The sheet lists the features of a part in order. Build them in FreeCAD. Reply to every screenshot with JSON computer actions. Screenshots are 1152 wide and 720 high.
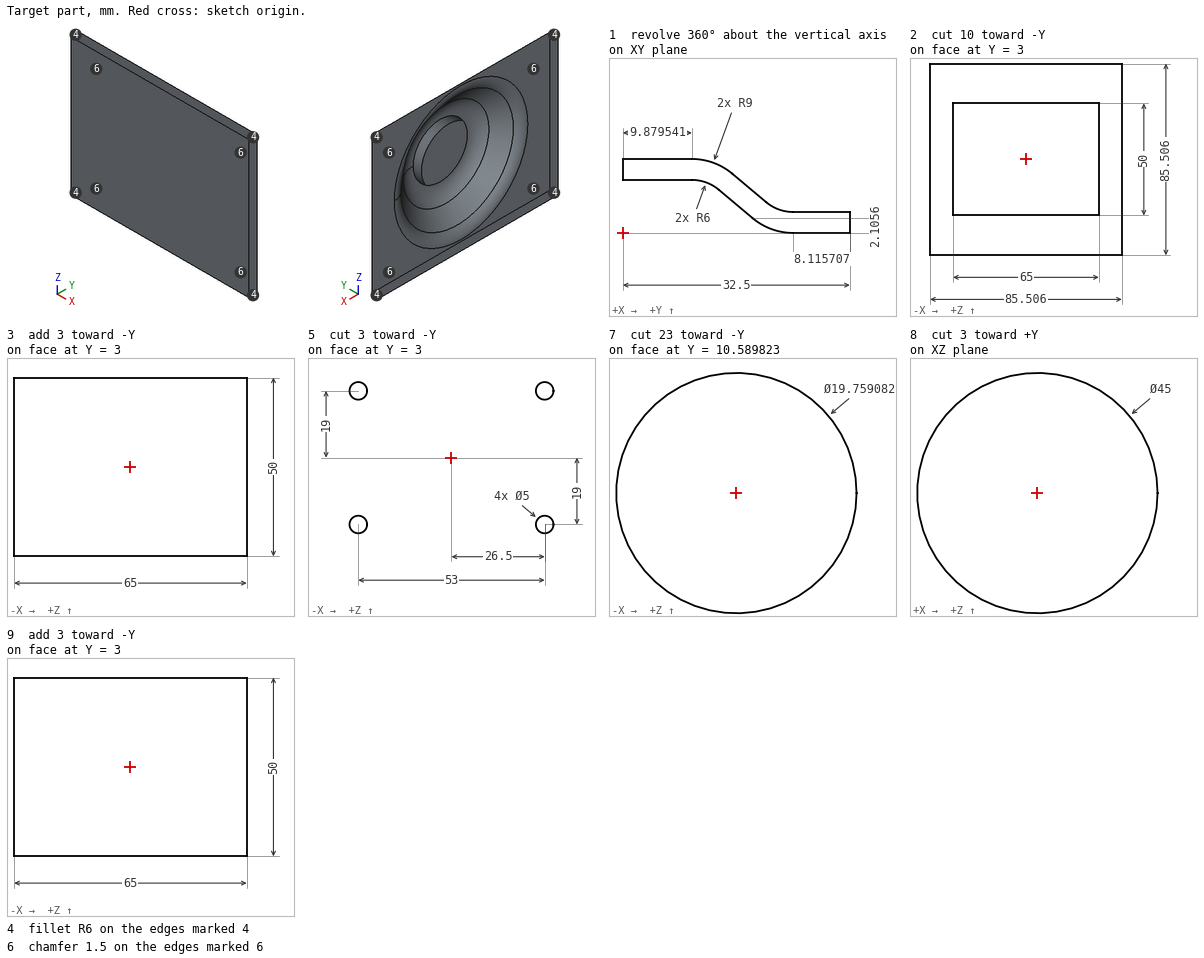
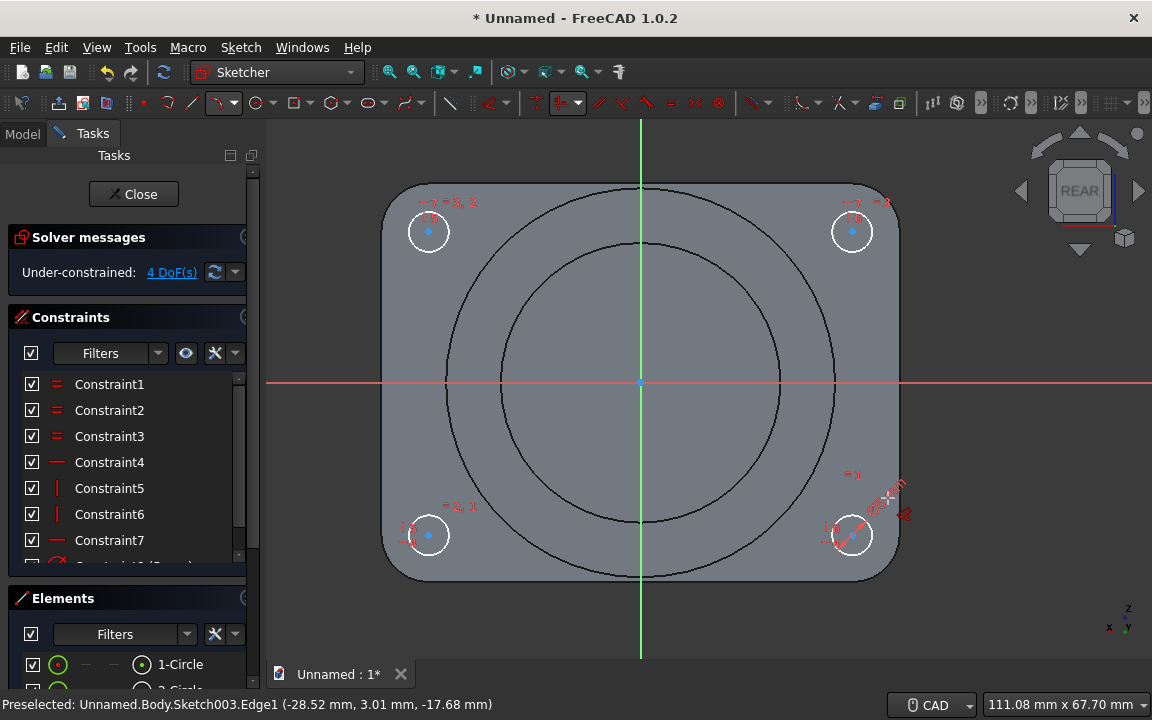
{"action": "left_click", "coordinate": [852, 535]}
{"action": "left_click", "coordinate": [886, 459]}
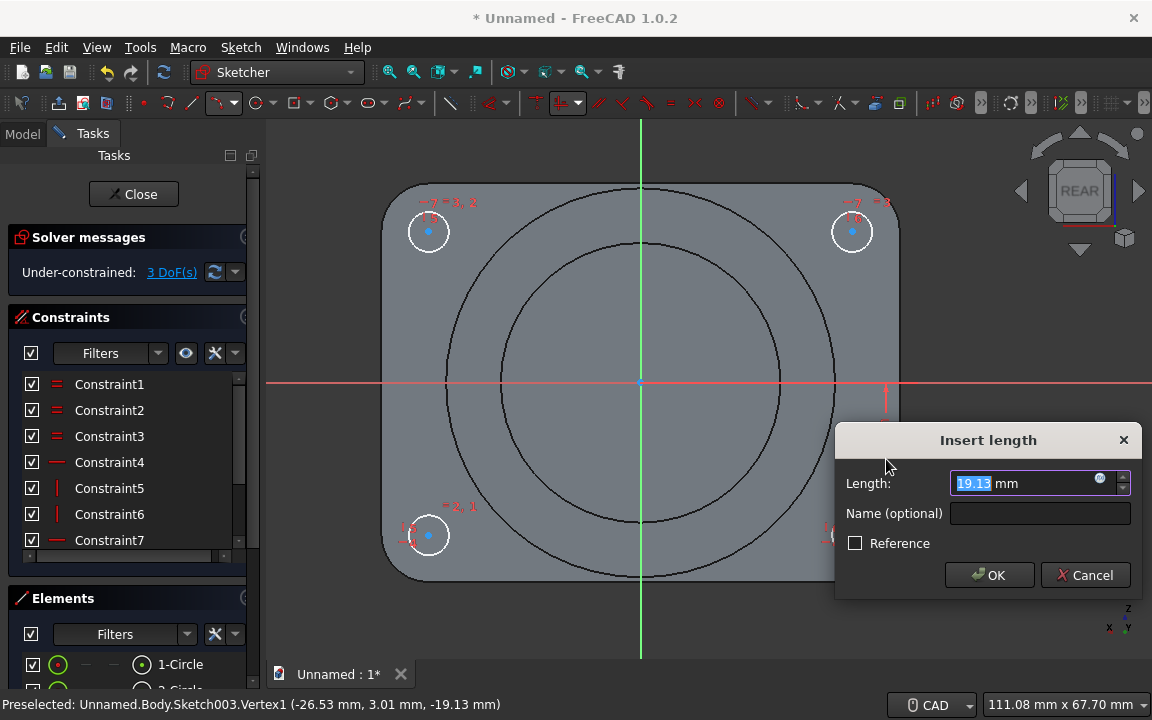
{"action": "type", "text": "19"}
{"action": "key", "text": "Return"}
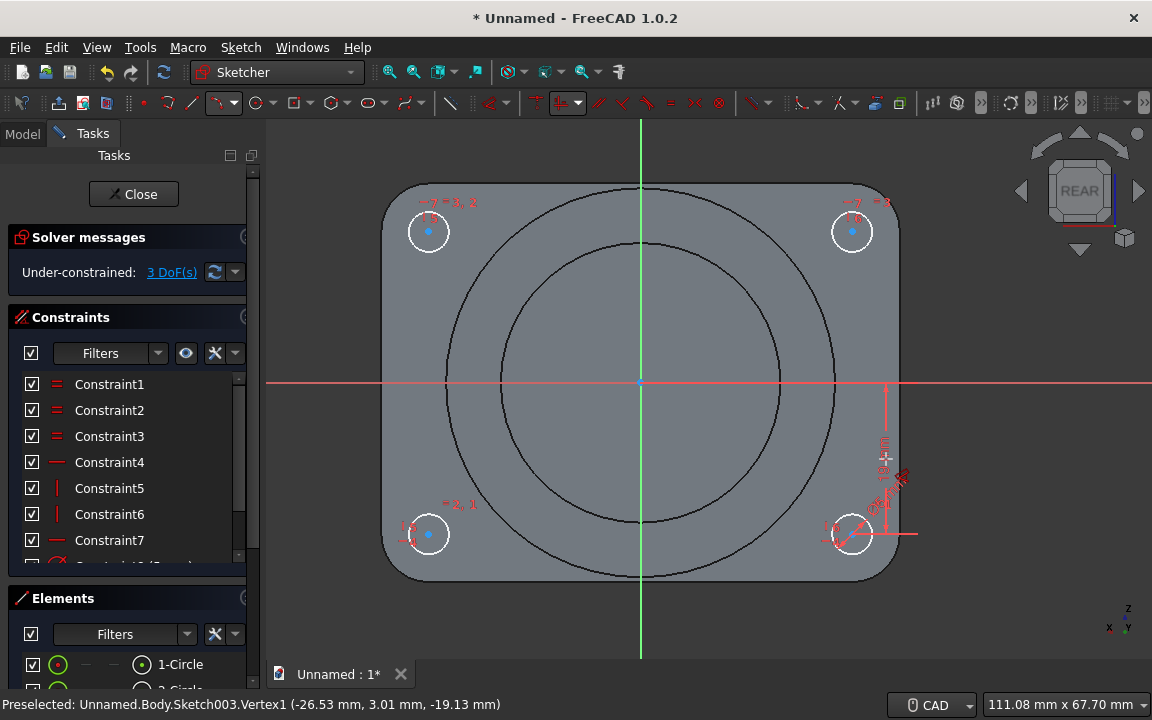
{"action": "left_click", "coordinate": [429, 232]}
{"action": "left_click", "coordinate": [395, 307]}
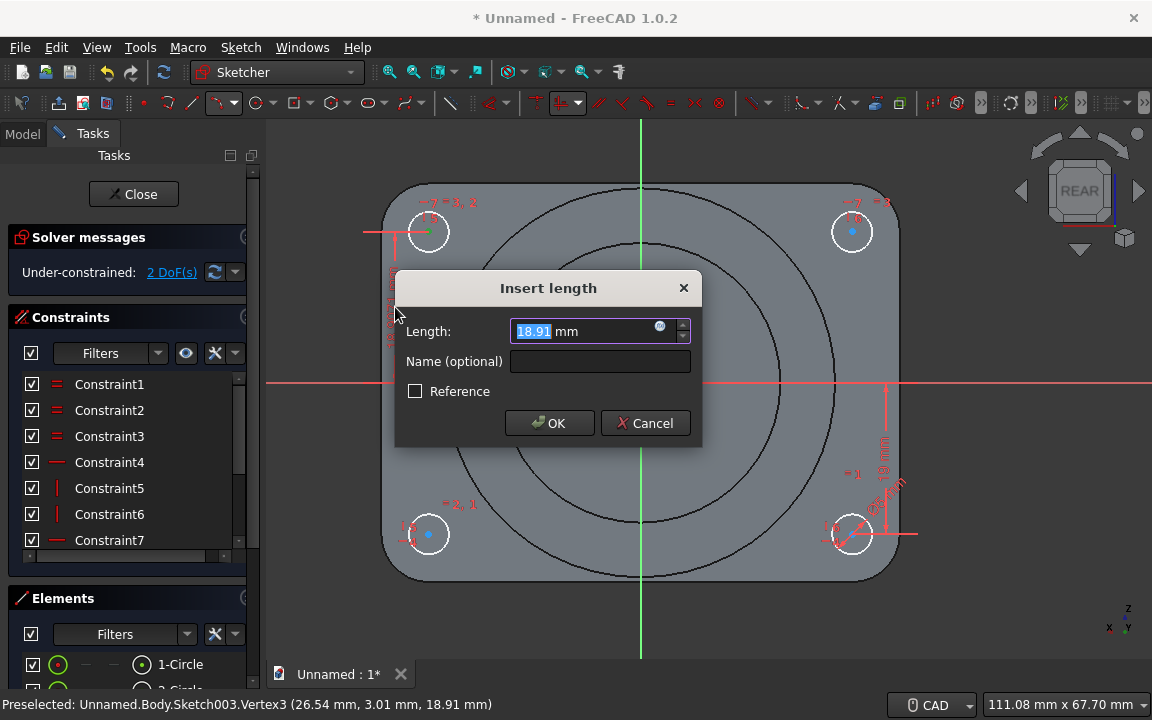
{"action": "type", "text": "19"}
{"action": "key", "text": "Return"}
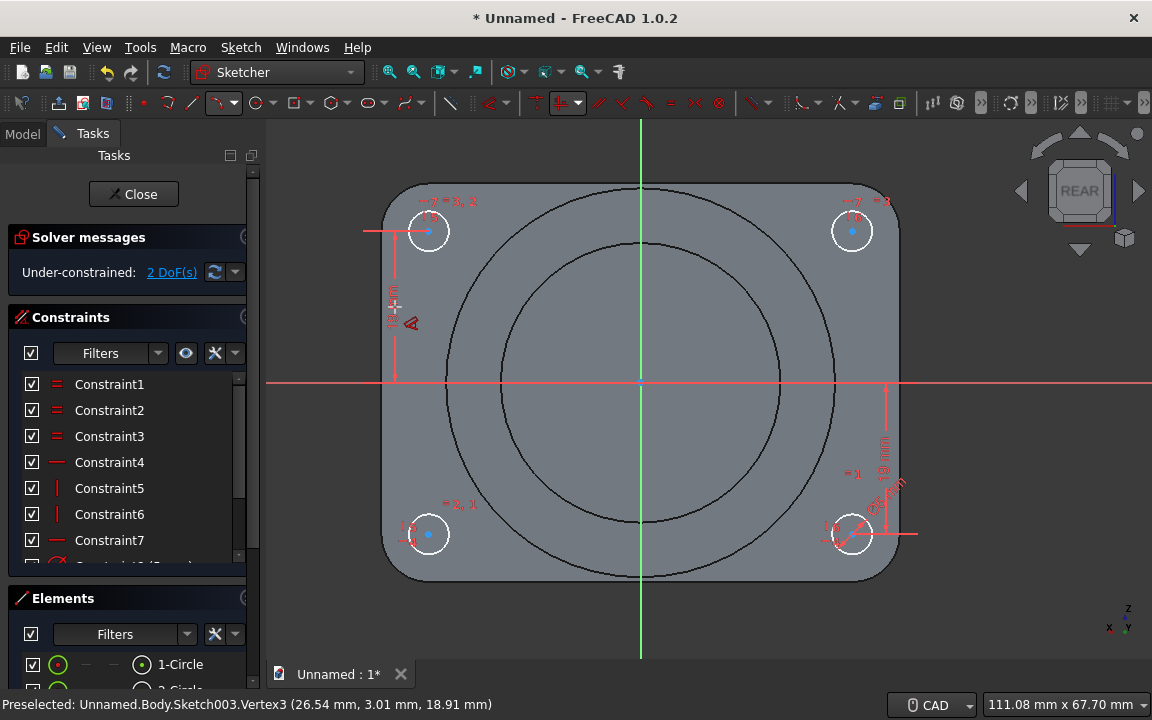
{"action": "left_click", "coordinate": [852, 534]}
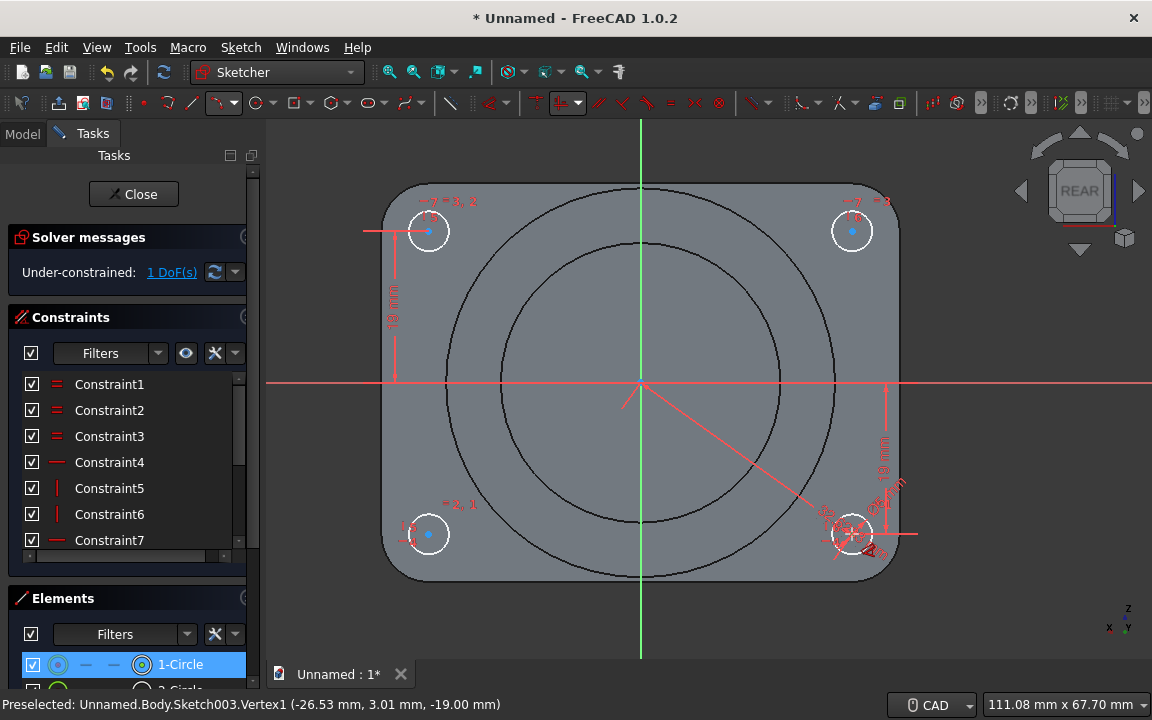
{"action": "left_click", "coordinate": [429, 534]}
{"action": "left_click", "coordinate": [543, 568]}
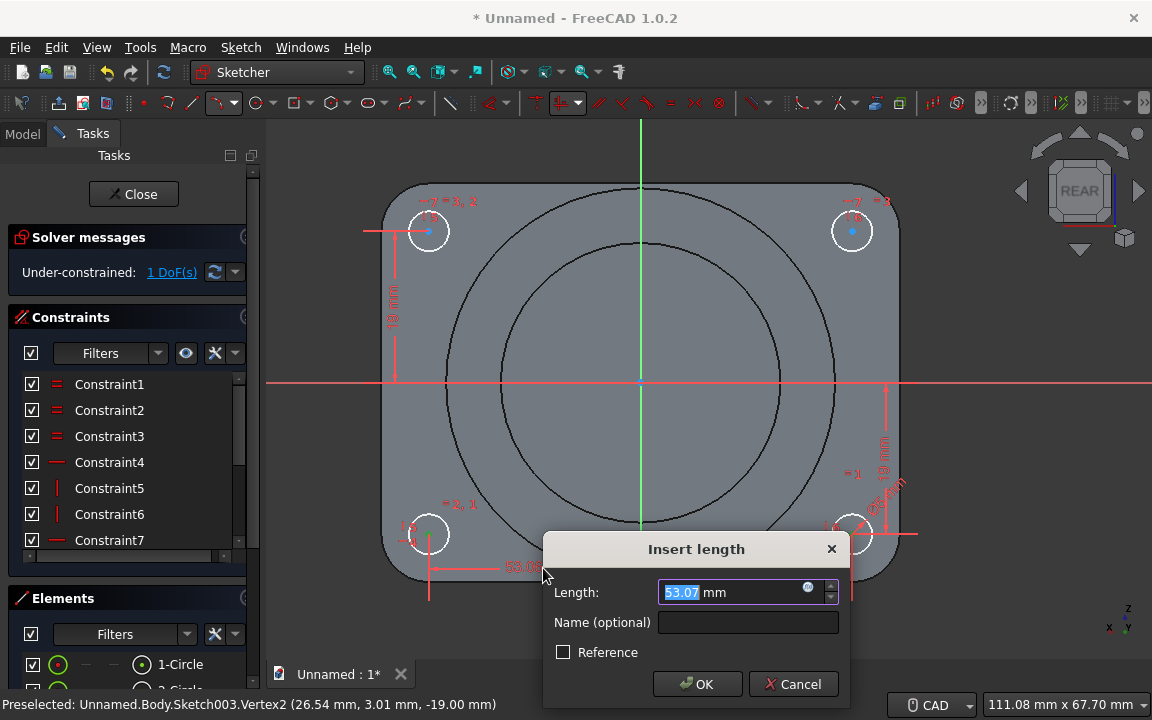
{"action": "type", "text": "53"}
{"action": "key", "text": "Return"}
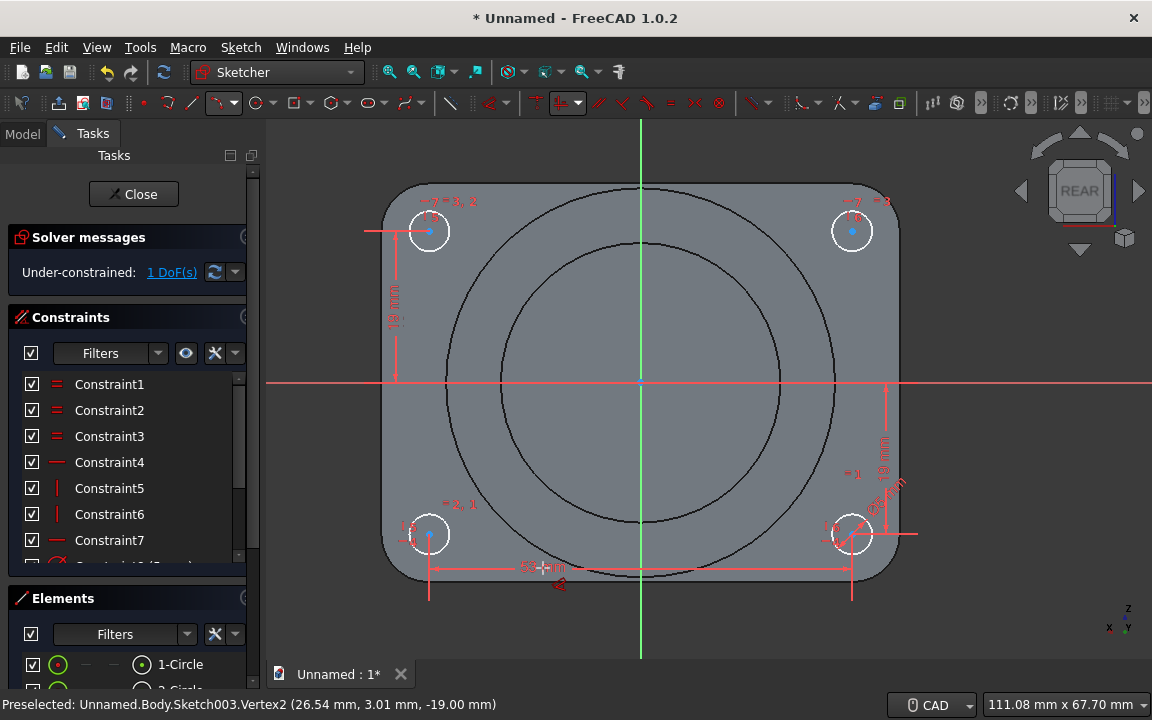
{"action": "left_click", "coordinate": [852, 534]}
{"action": "left_click", "coordinate": [746, 568]}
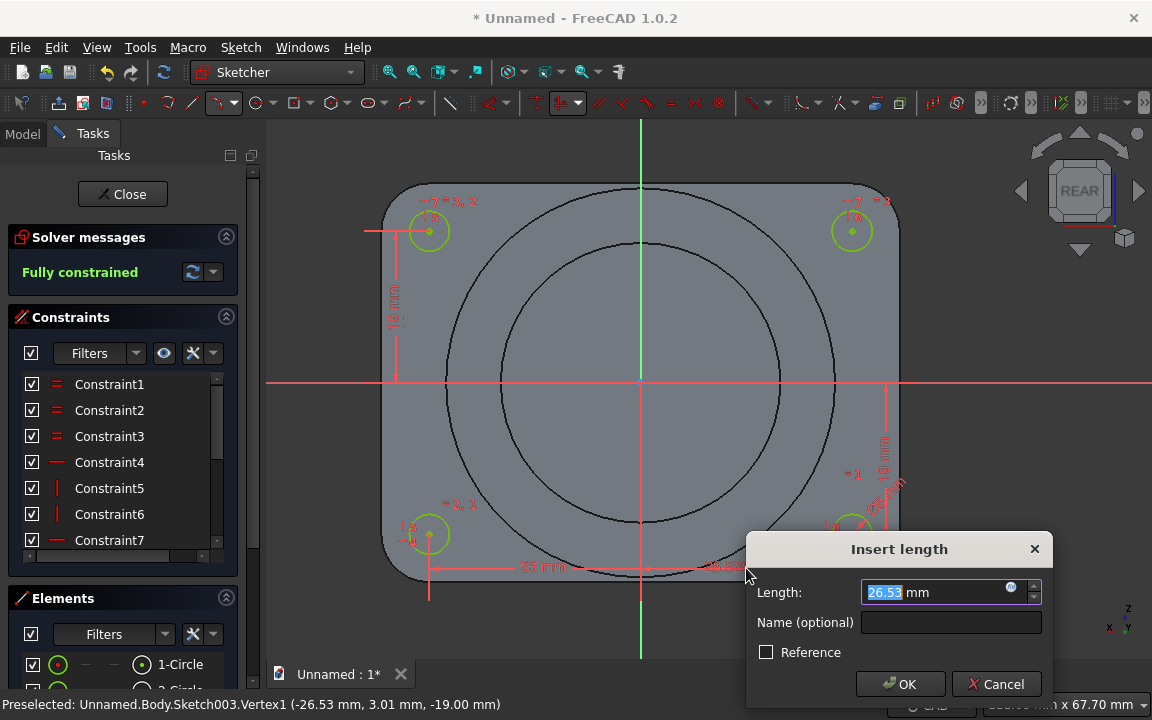
{"action": "type", "text": "26.5"}
{"action": "key", "text": "Return"}
{"action": "key", "text": "Escape"}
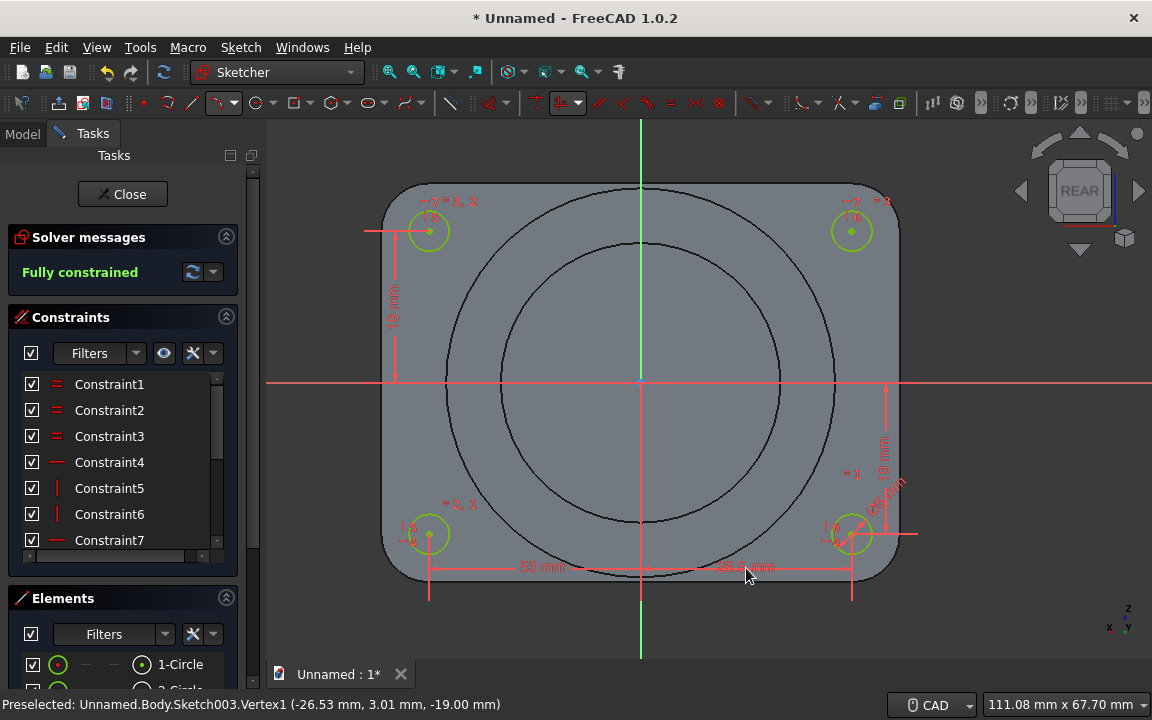
{"action": "left_click", "coordinate": [123, 194]}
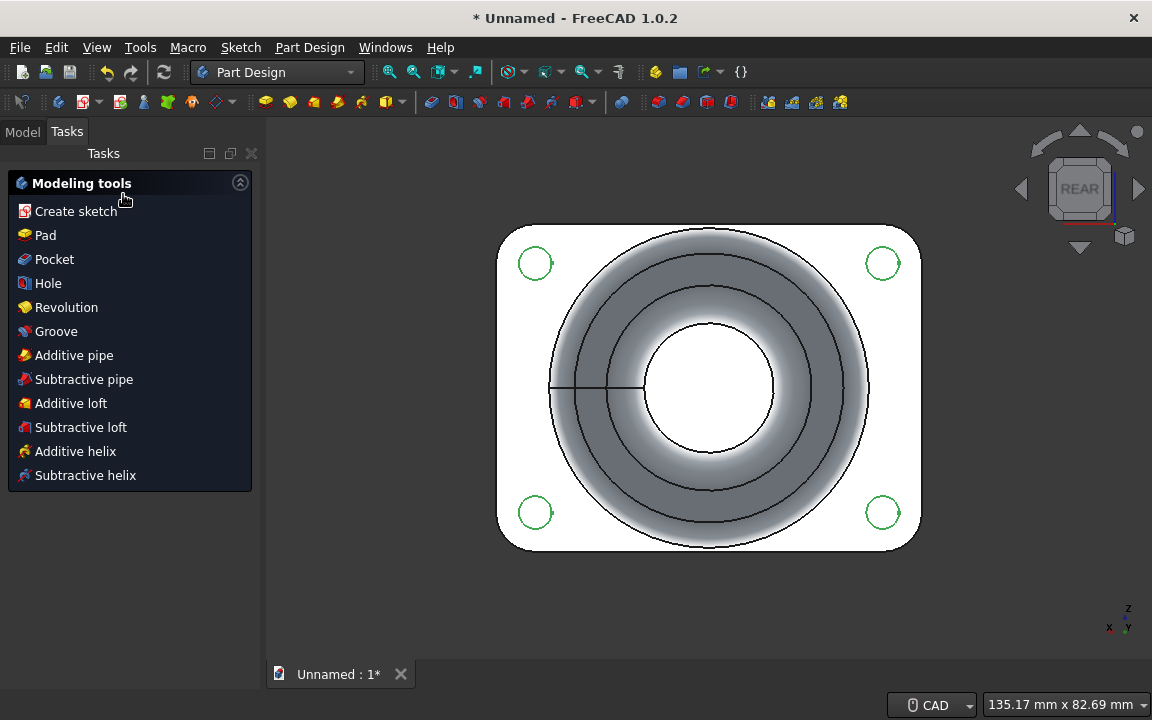
{"action": "left_click", "coordinate": [432, 102]}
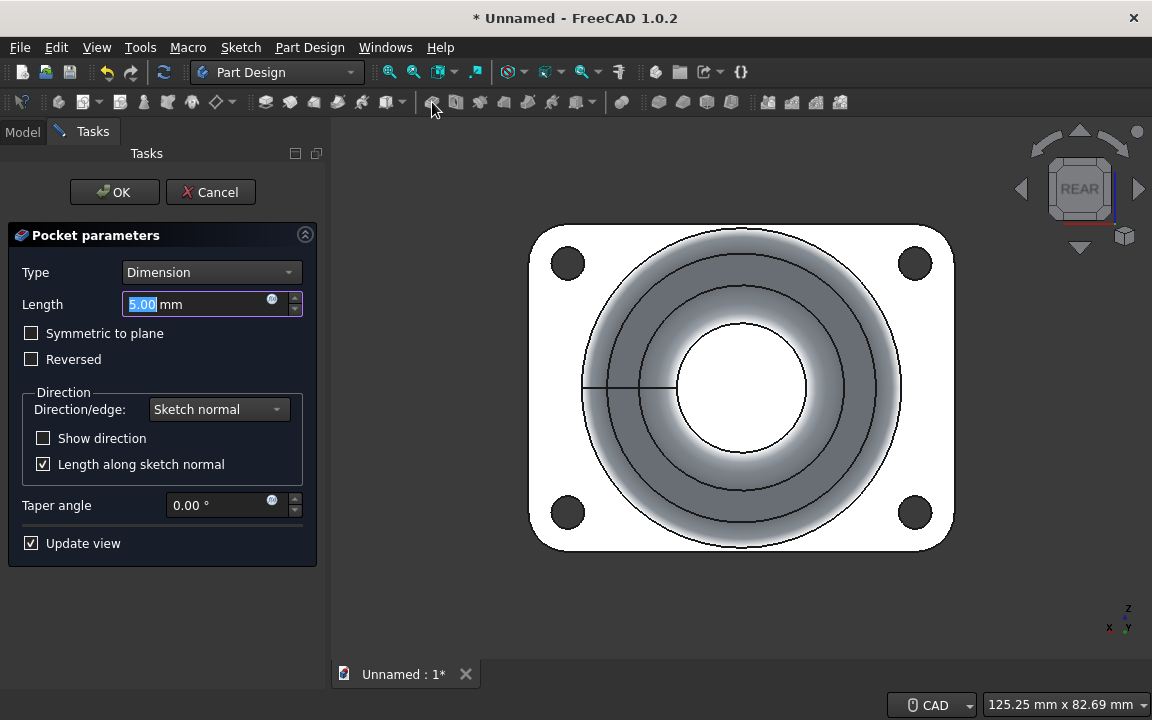
{"action": "type", "text": "3"}
{"action": "key", "text": "Tab"}